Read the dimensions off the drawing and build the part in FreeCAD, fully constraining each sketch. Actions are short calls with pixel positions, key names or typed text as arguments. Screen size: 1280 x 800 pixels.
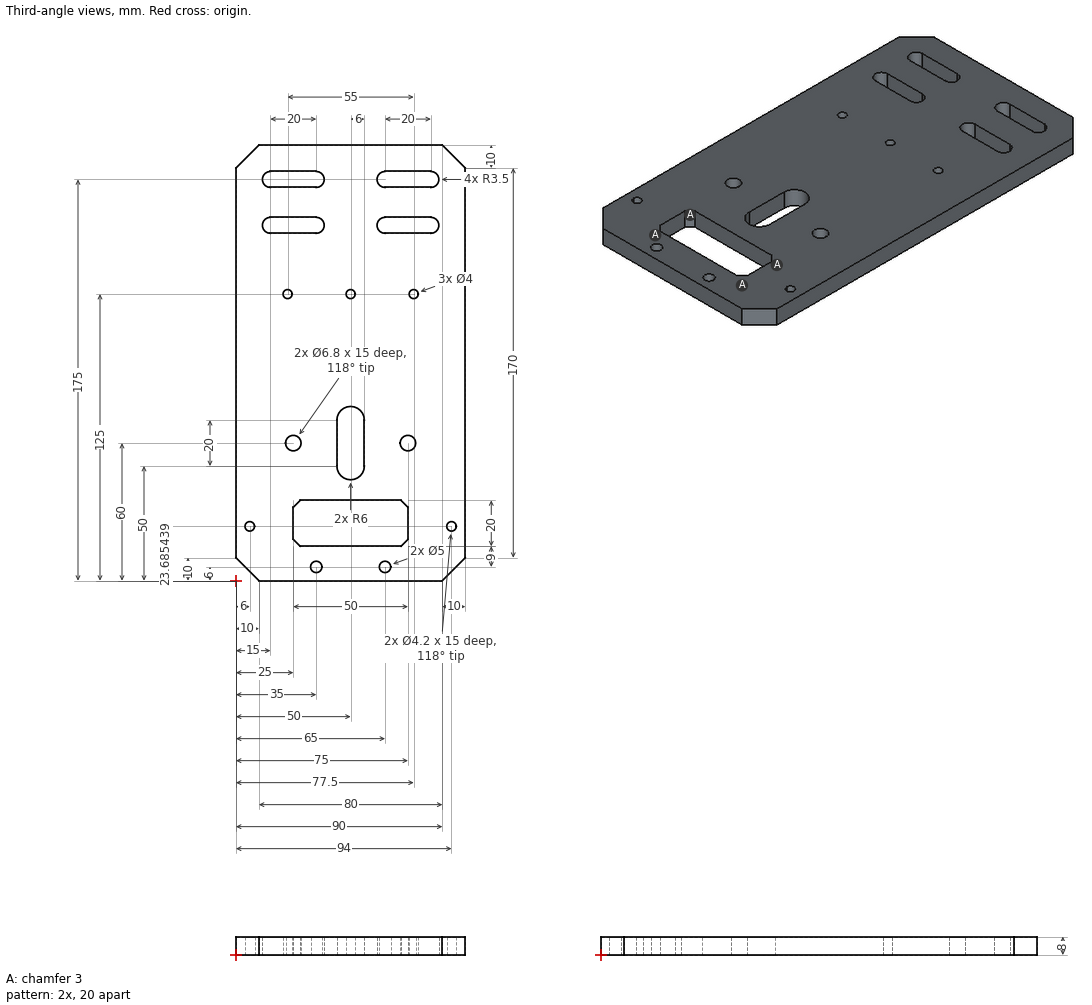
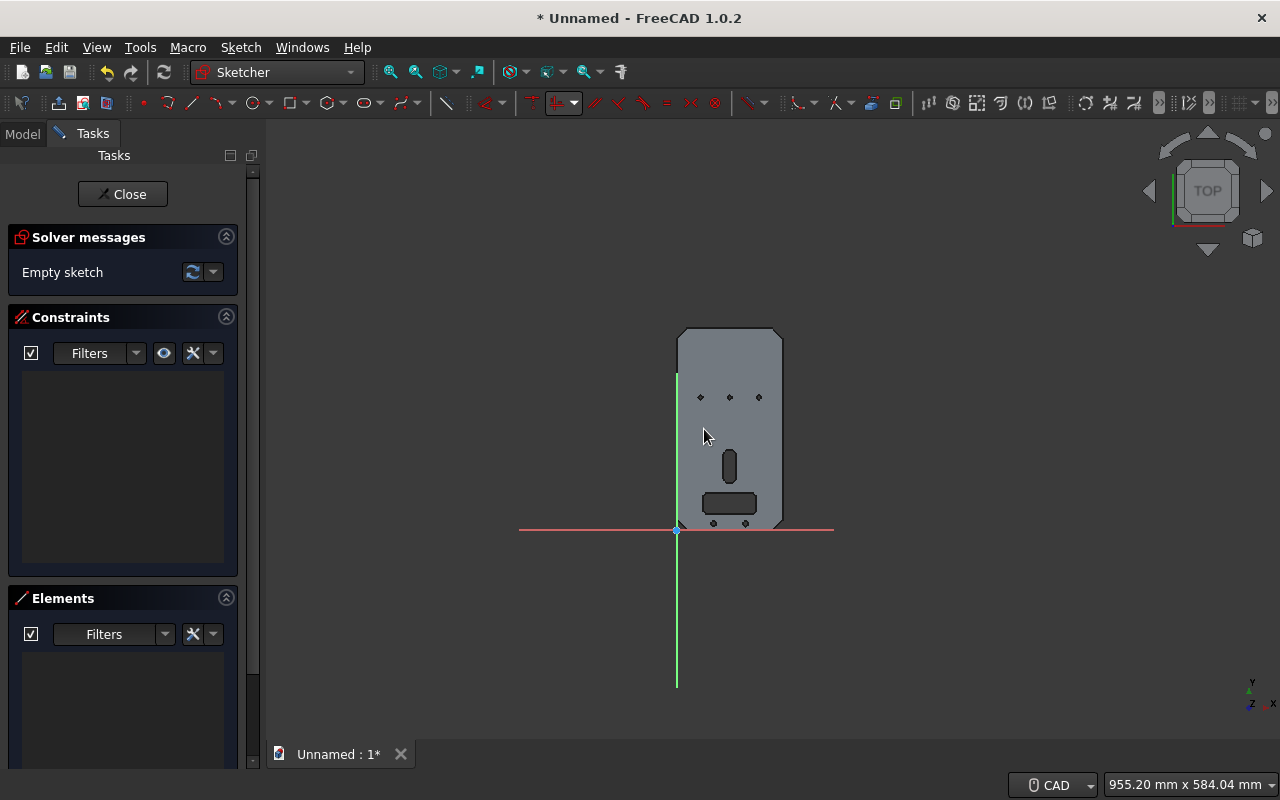
scroll(721, 510, up, 9)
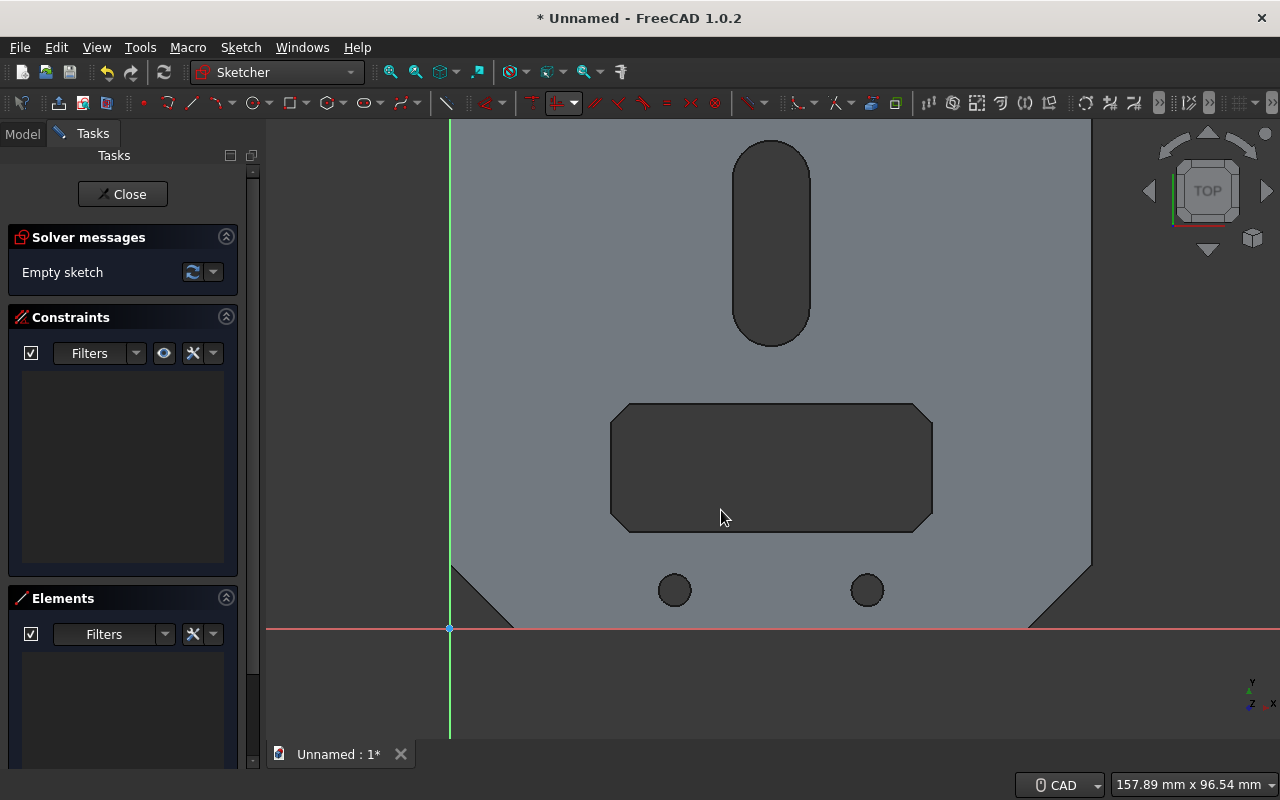
key(g)
key(c)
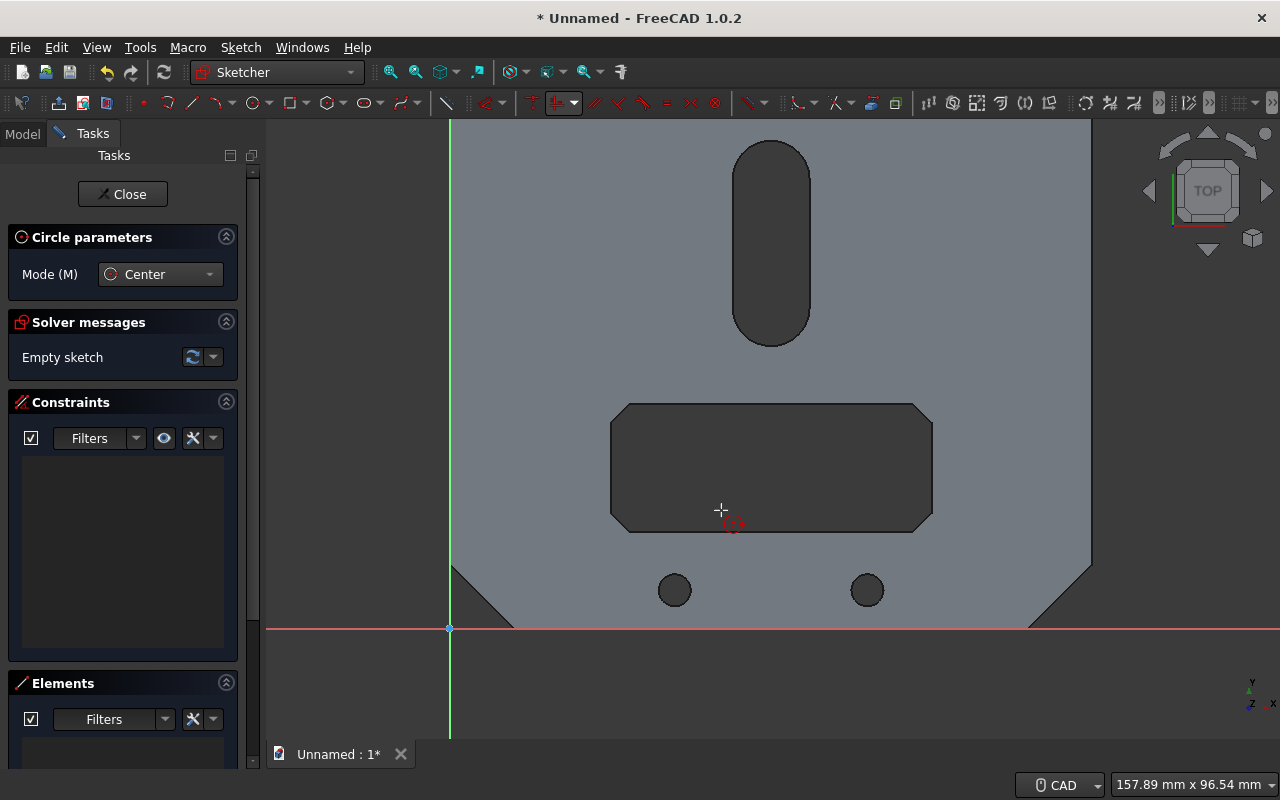
click(611, 243)
move(626, 228)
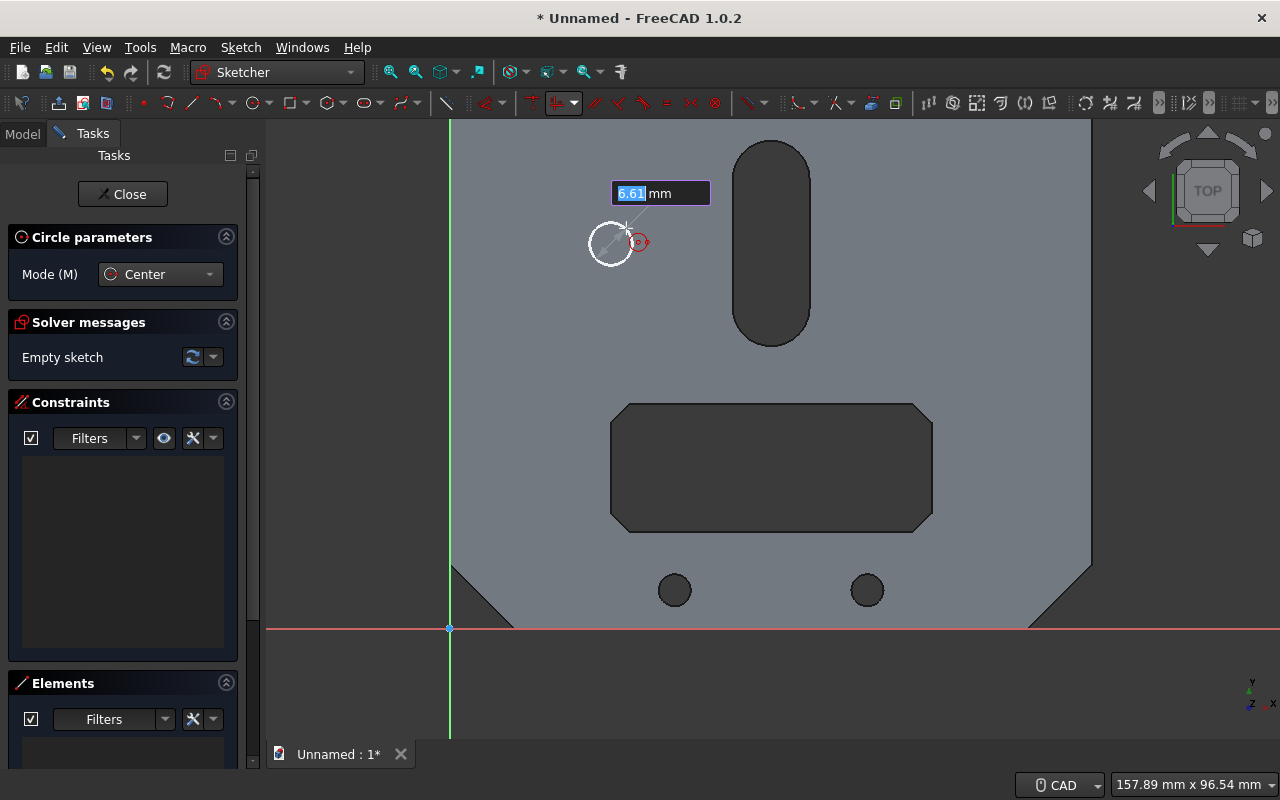
text(6.8)
key(Return)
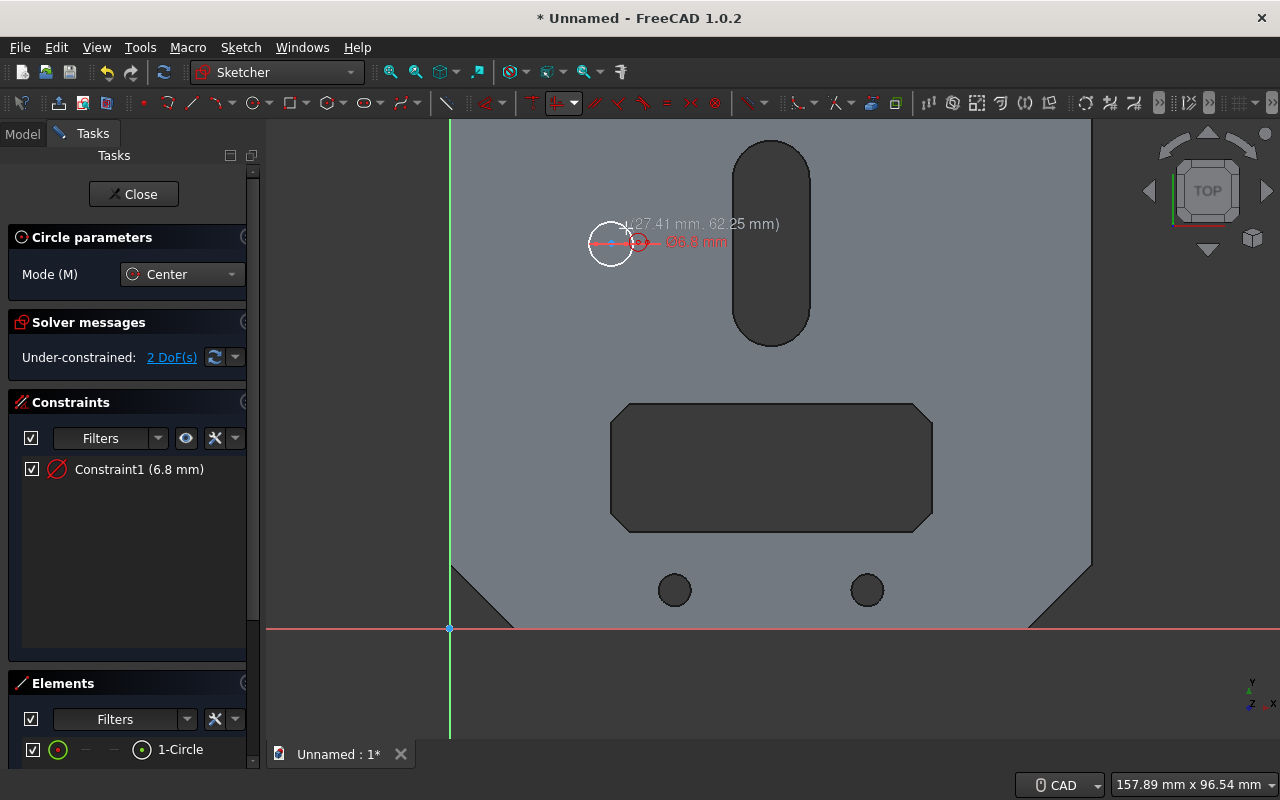
click(932, 243)
move(947, 228)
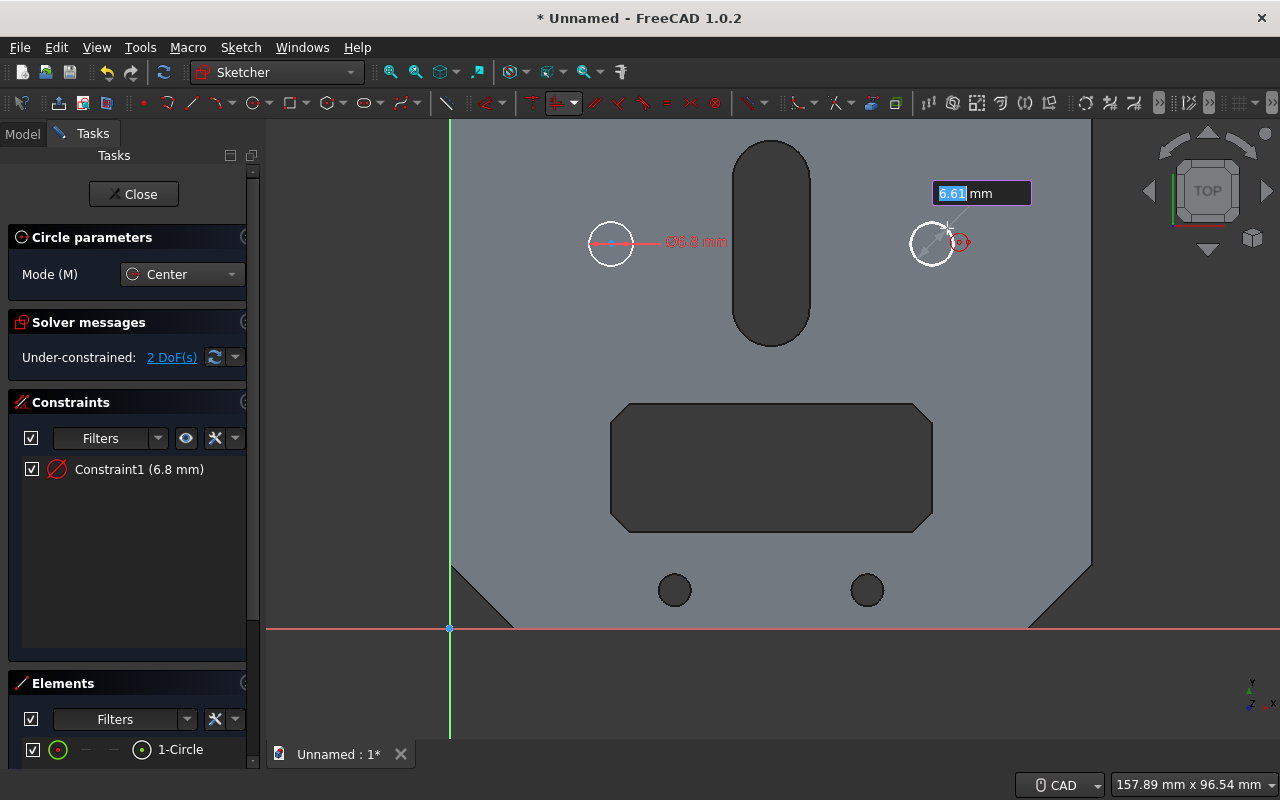
text(6.8)
key(Return)
key(Escape)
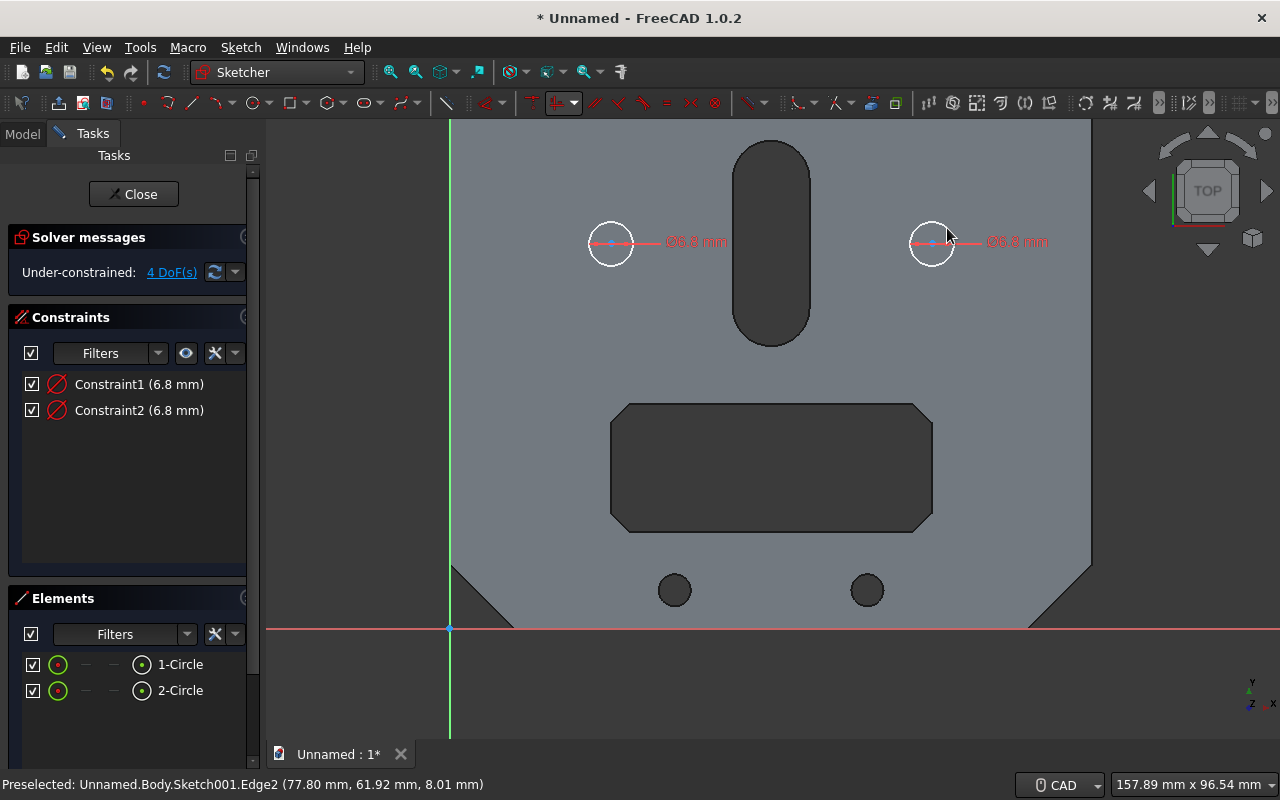
click(611, 244)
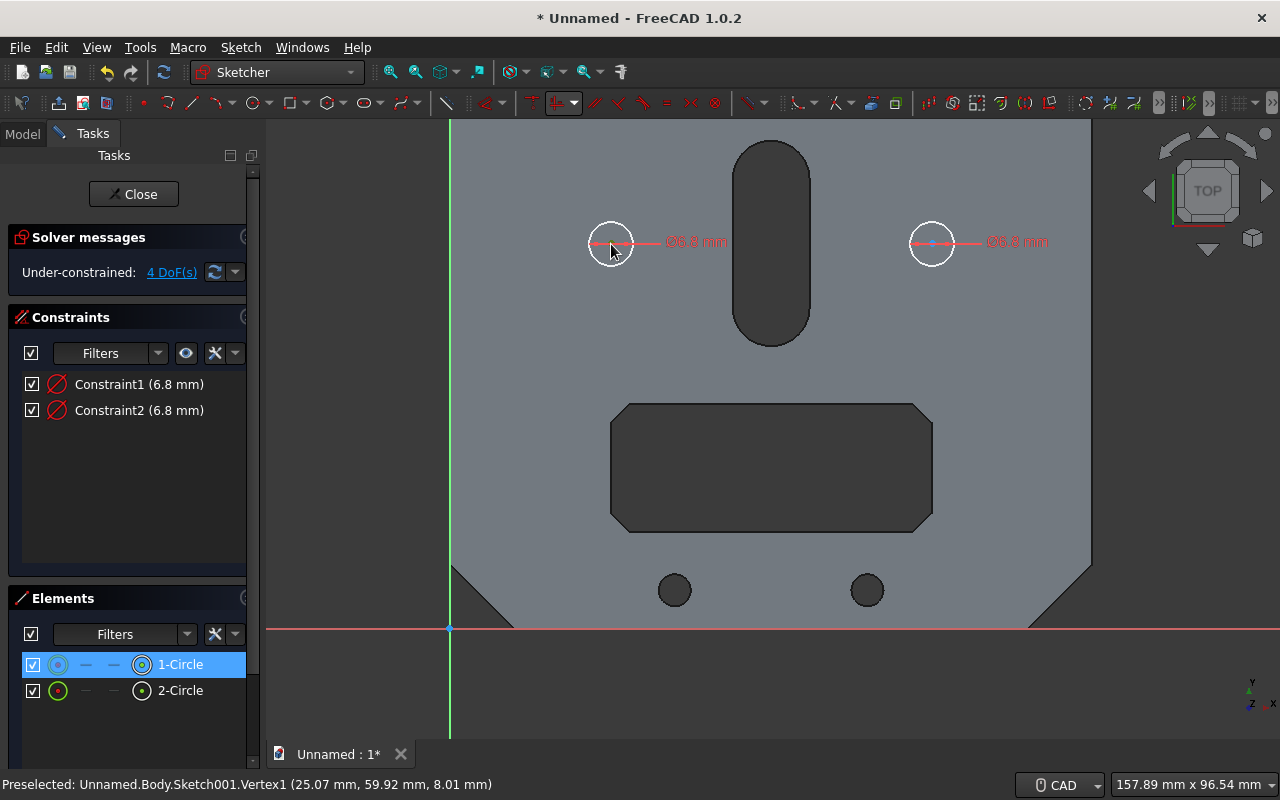
click(932, 244)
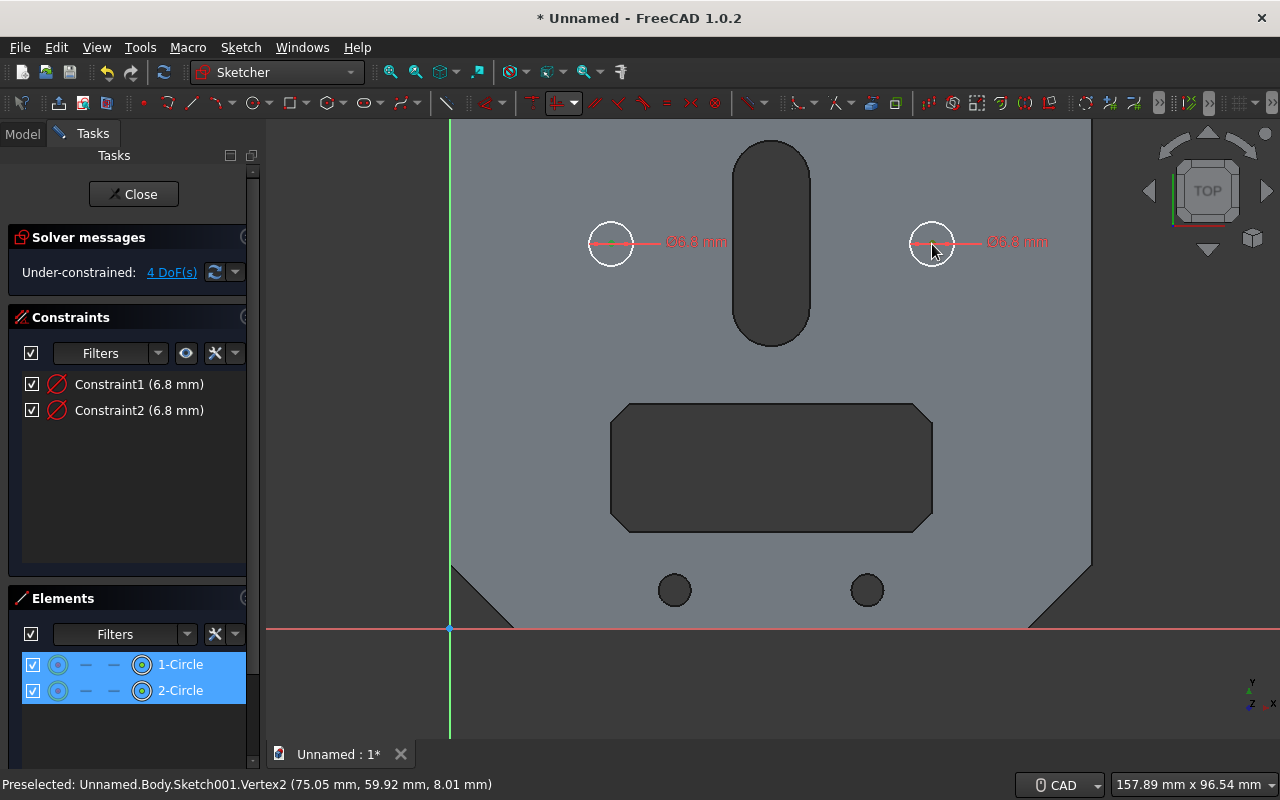
click(576, 104)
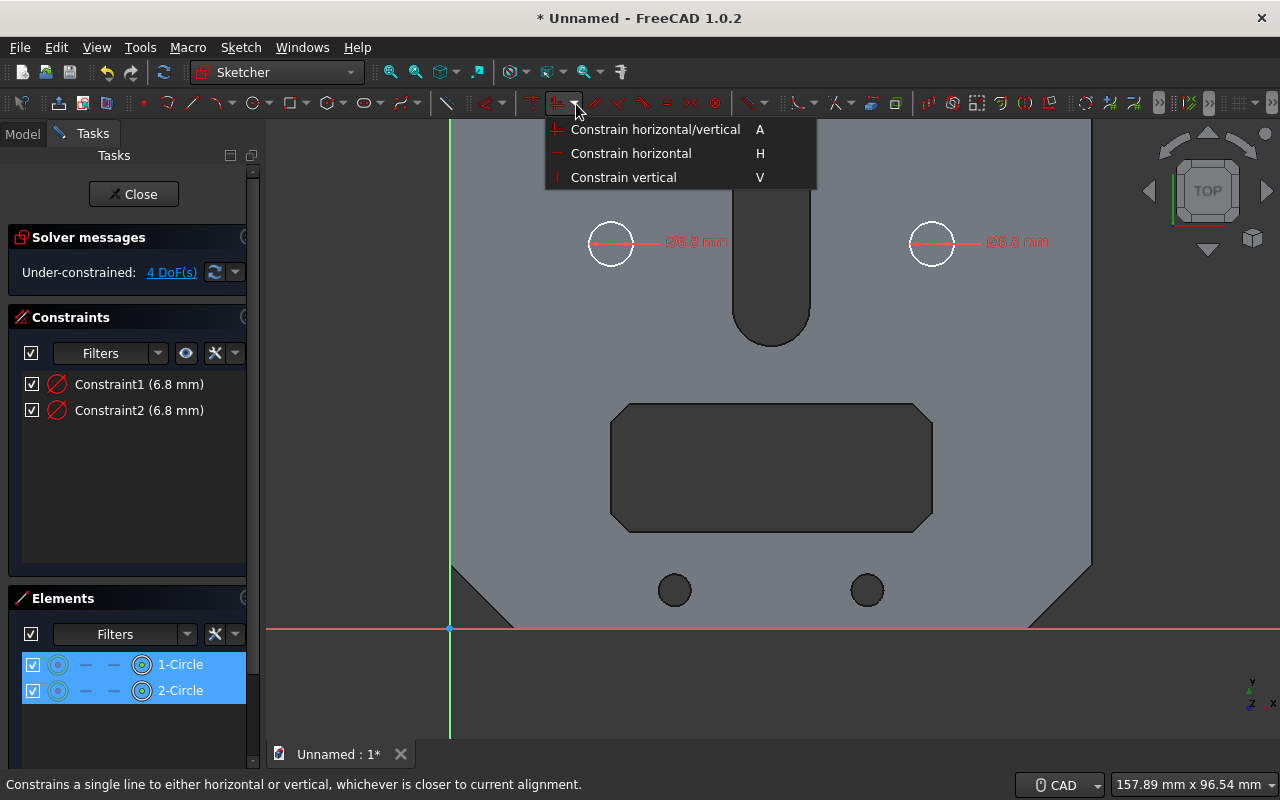
click(681, 153)